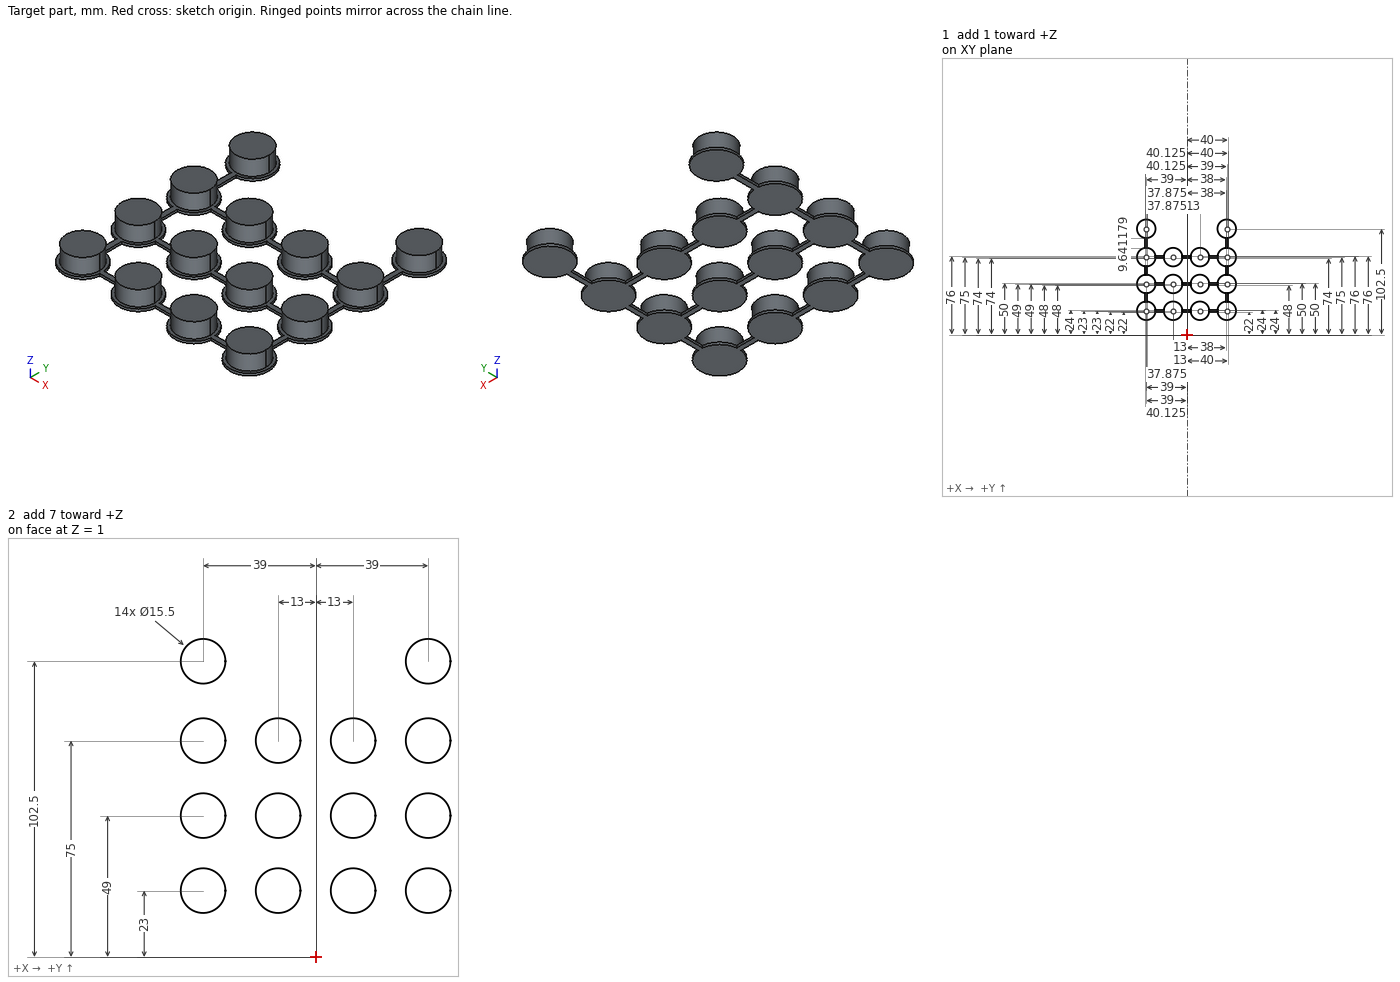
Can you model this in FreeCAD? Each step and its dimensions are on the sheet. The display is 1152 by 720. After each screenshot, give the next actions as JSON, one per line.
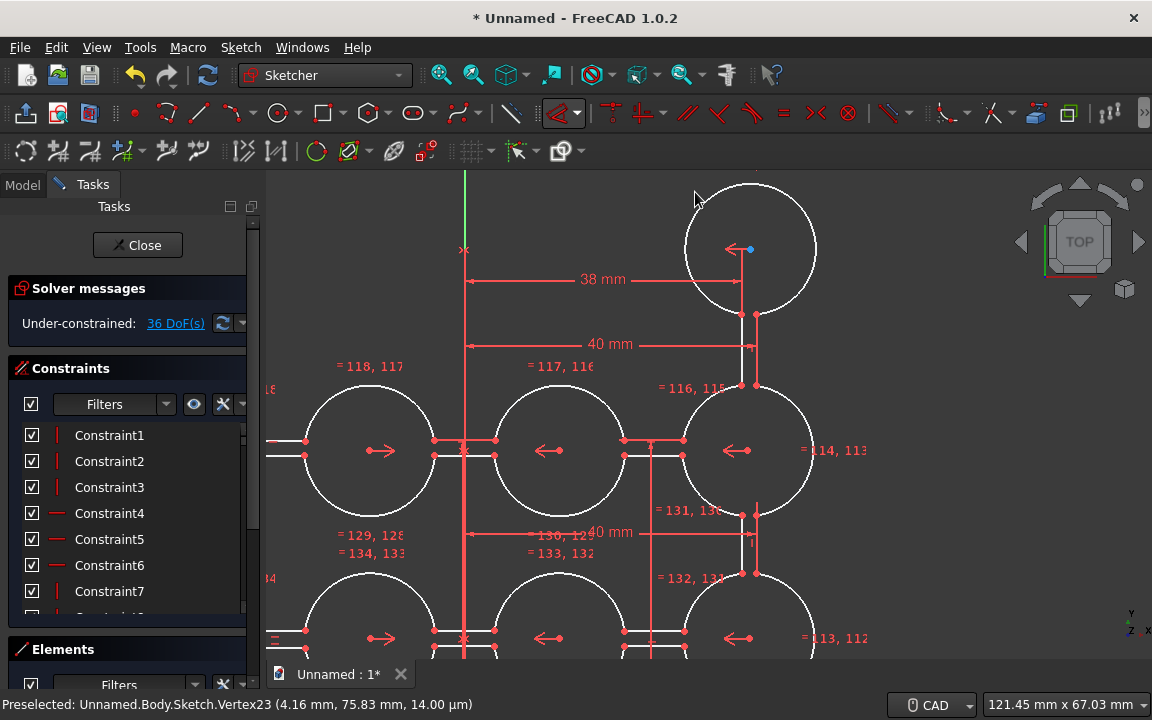
{"action": "left_click", "coordinate": [305, 441]}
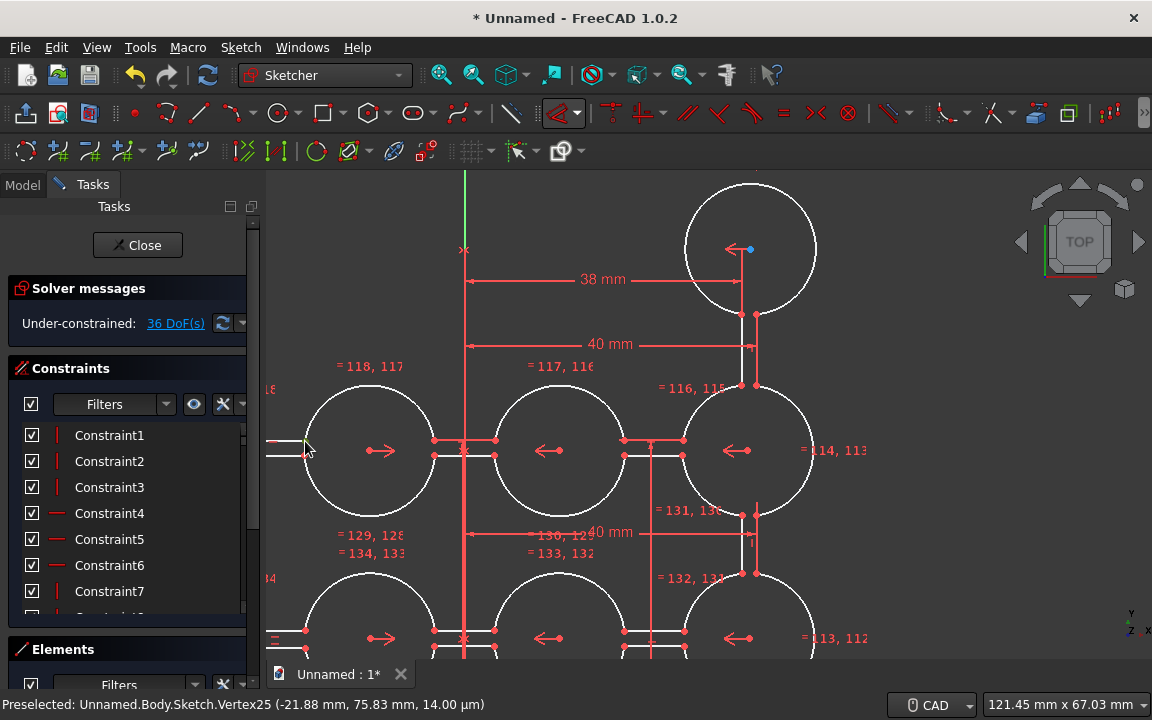
{"action": "left_click", "coordinate": [580, 114]}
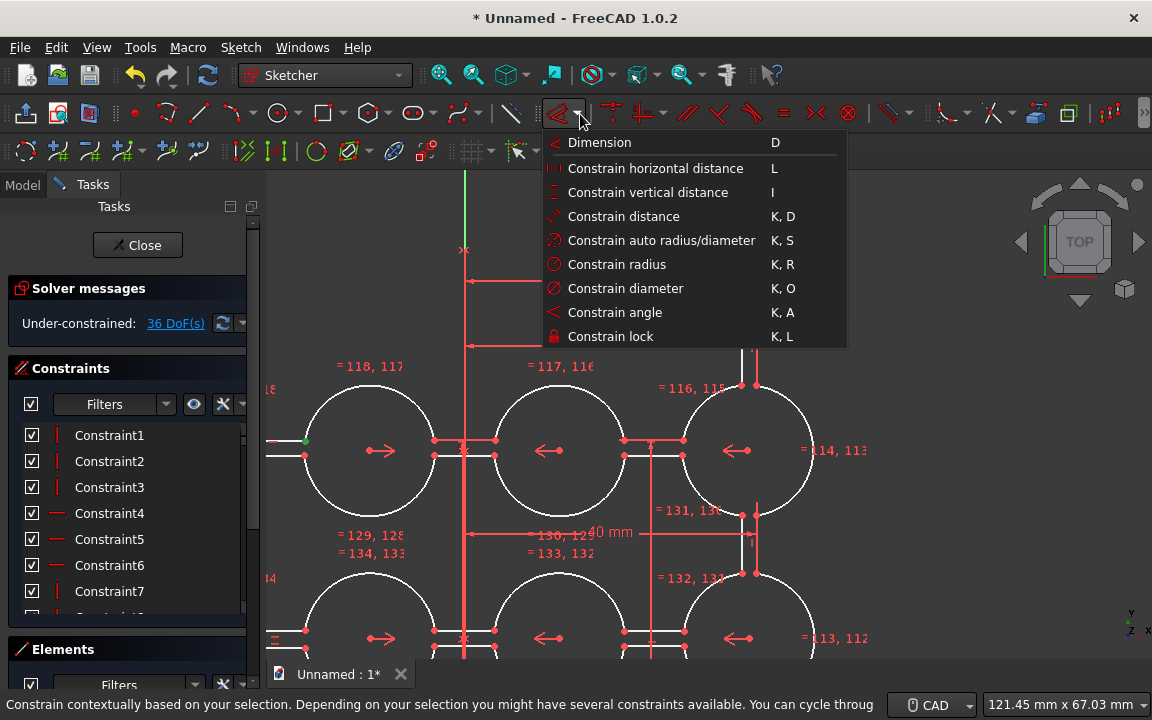
{"action": "left_click", "coordinate": [695, 192]}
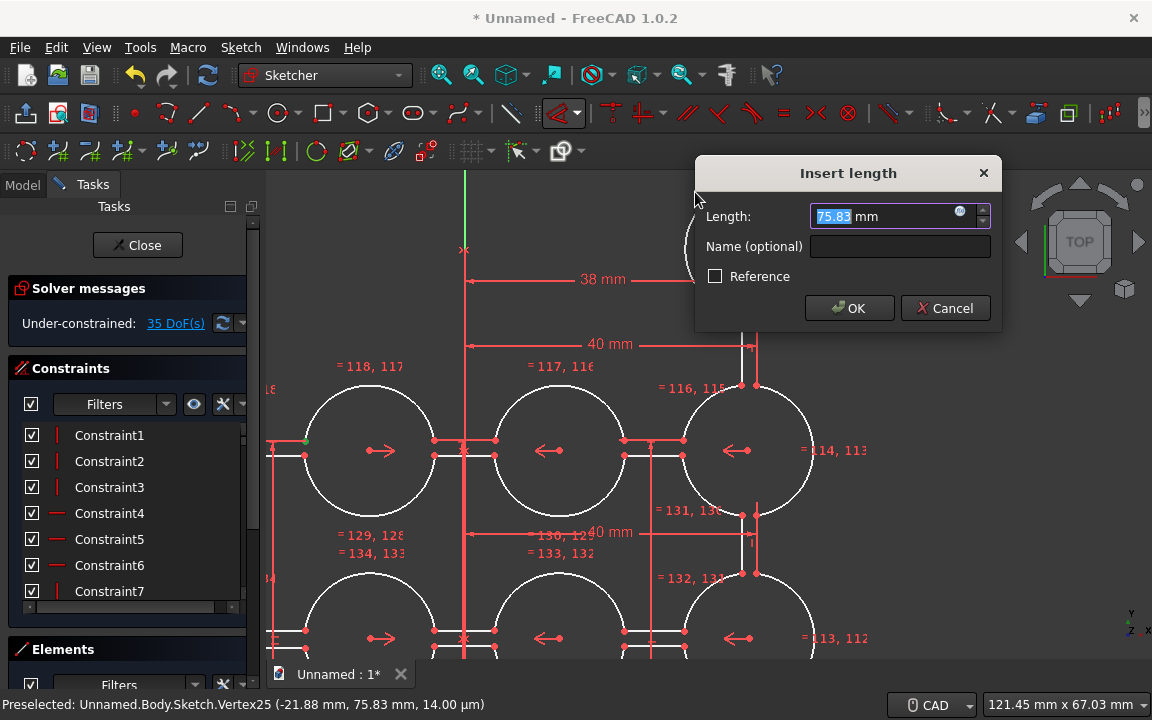
{"action": "type", "text": "76"}
{"action": "key", "text": "Return"}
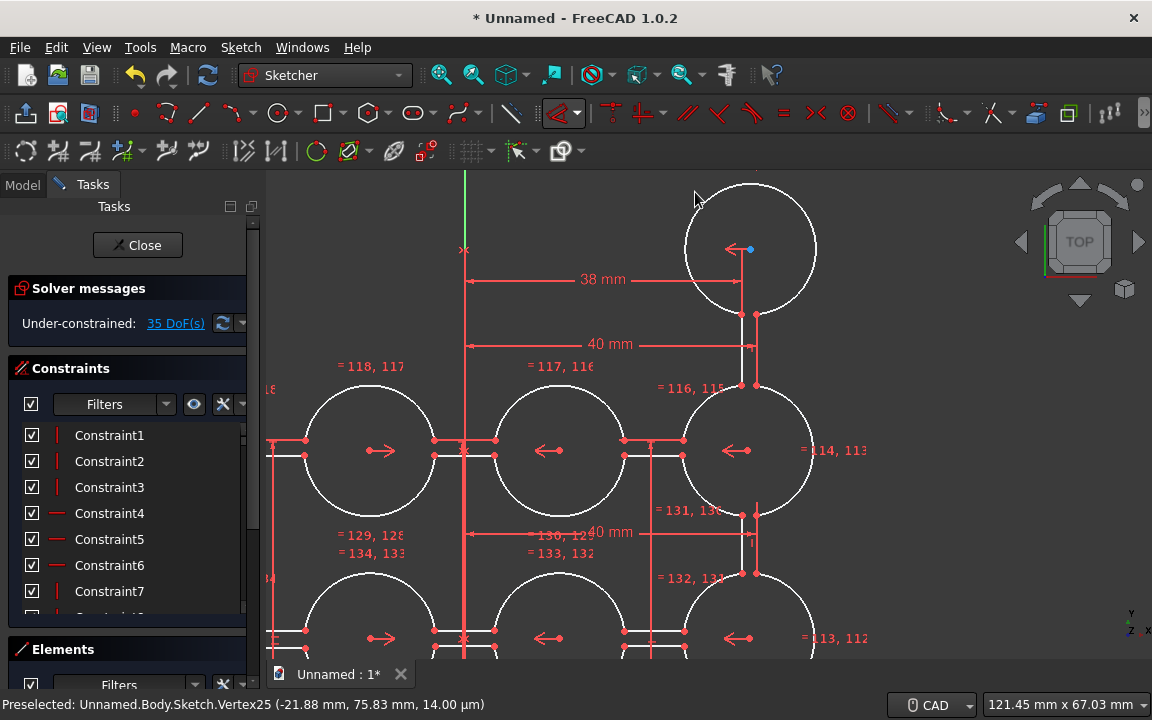
{"action": "scroll", "coordinate": [743, 314], "scroll_direction": "down", "scroll_amount": 5}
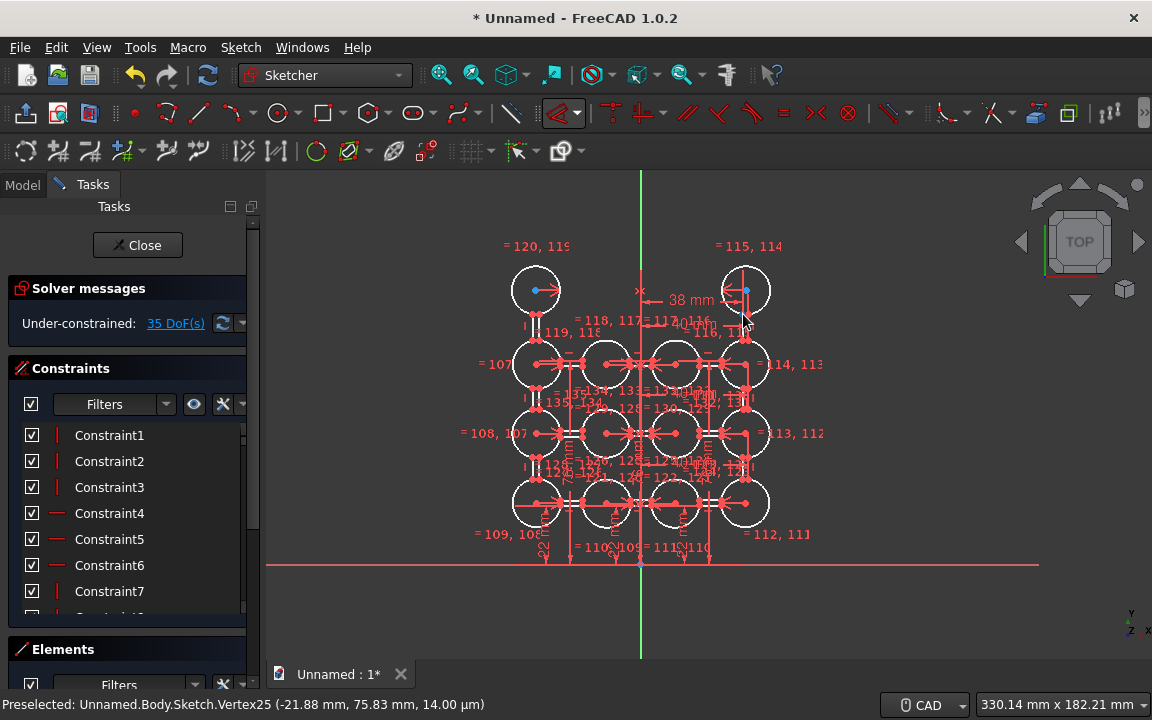
{"action": "scroll", "coordinate": [560, 437], "scroll_direction": "up", "scroll_amount": 4}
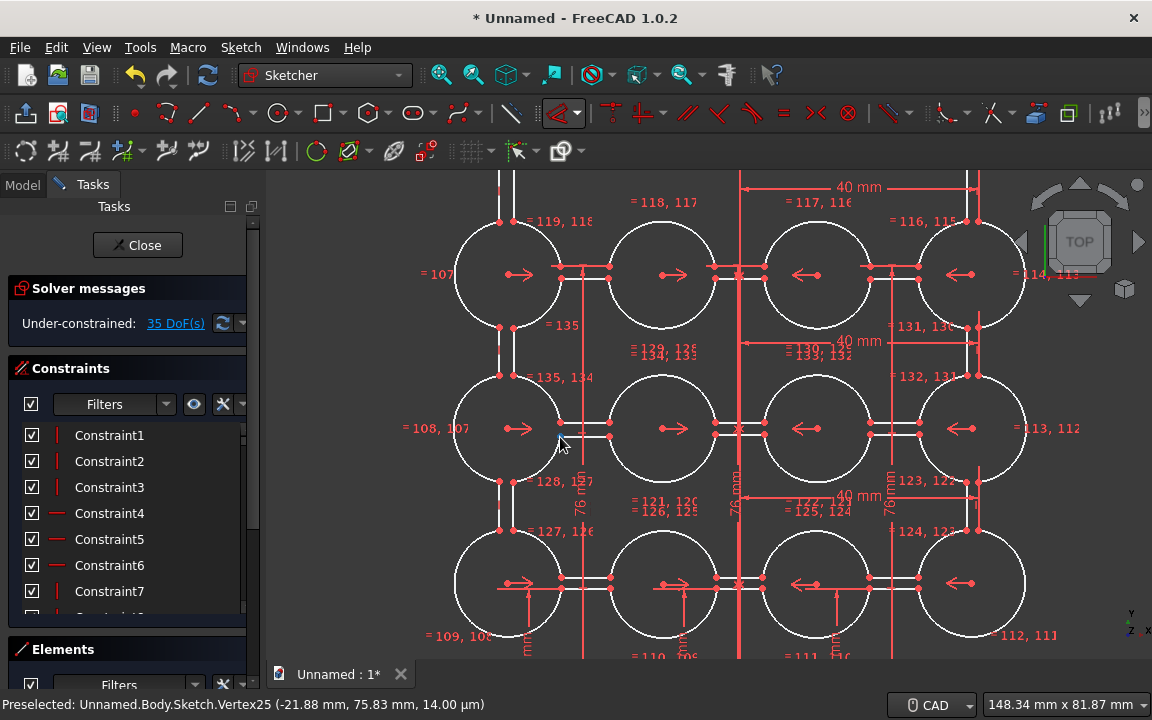
{"action": "left_click", "coordinate": [560, 437]}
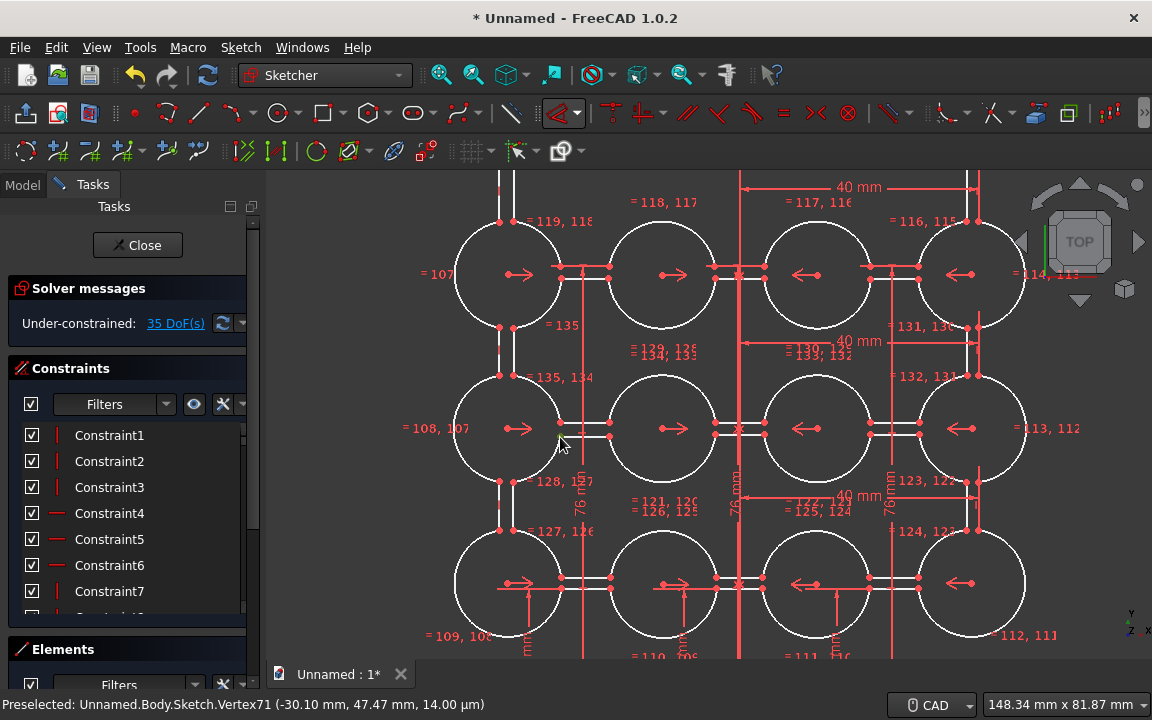
{"action": "left_click", "coordinate": [580, 114]}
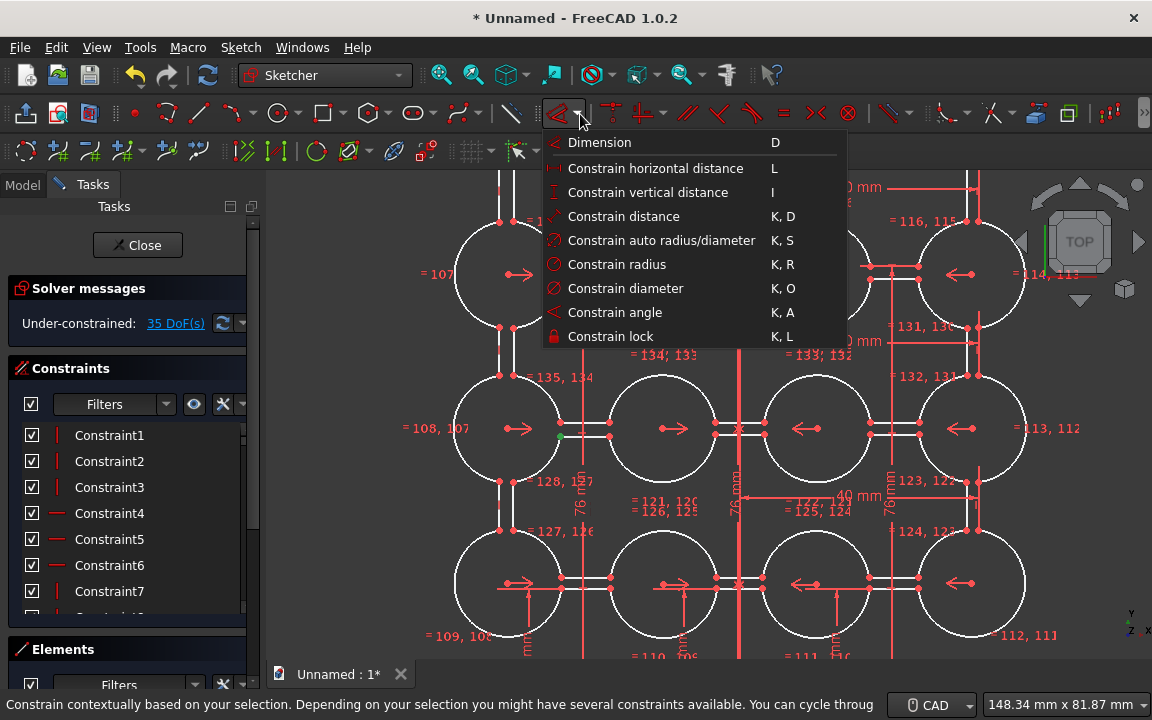
{"action": "left_click", "coordinate": [695, 192]}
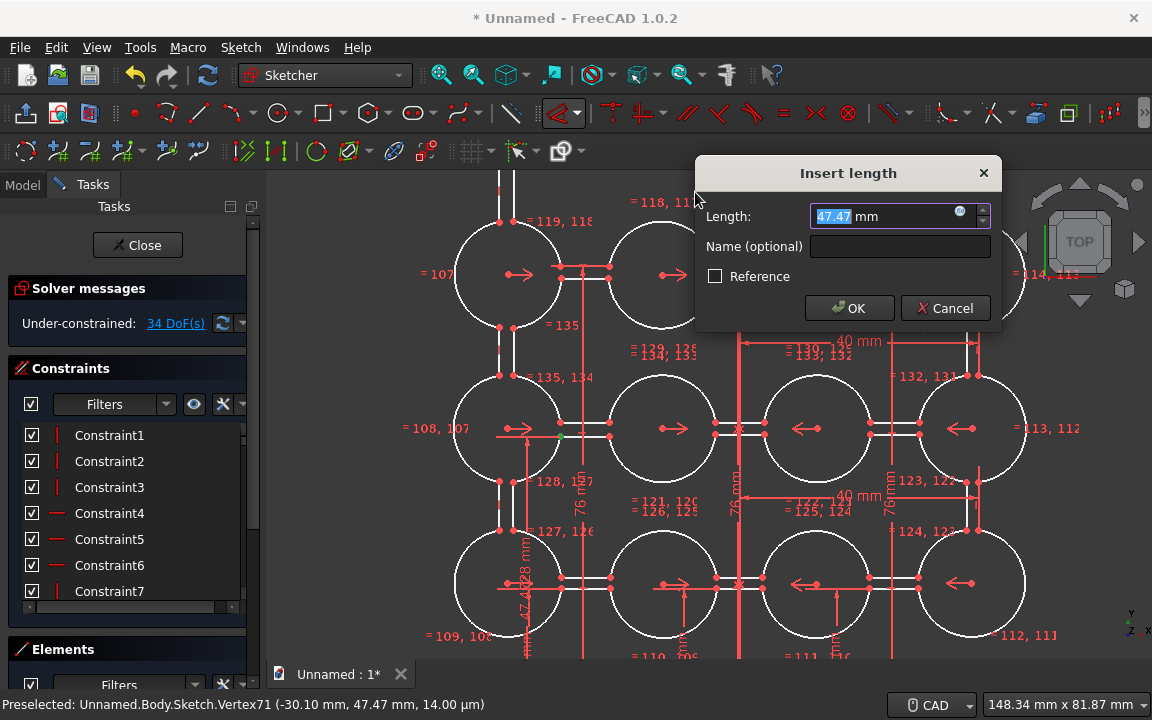
{"action": "type", "text": "48"}
{"action": "key", "text": "Return"}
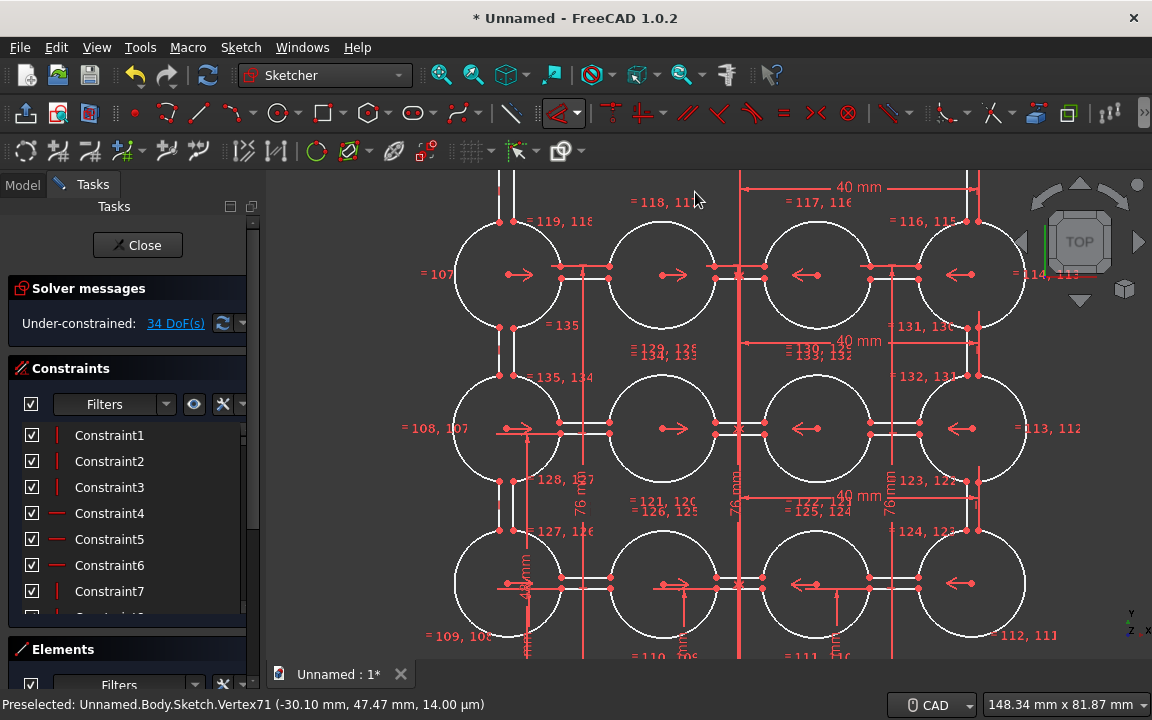
{"action": "left_click", "coordinate": [715, 435]}